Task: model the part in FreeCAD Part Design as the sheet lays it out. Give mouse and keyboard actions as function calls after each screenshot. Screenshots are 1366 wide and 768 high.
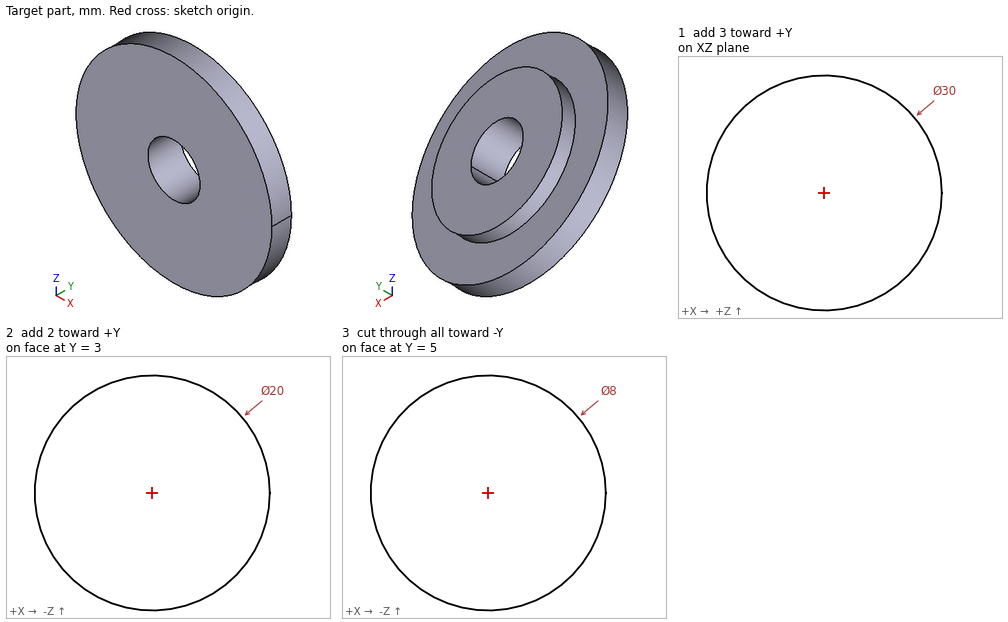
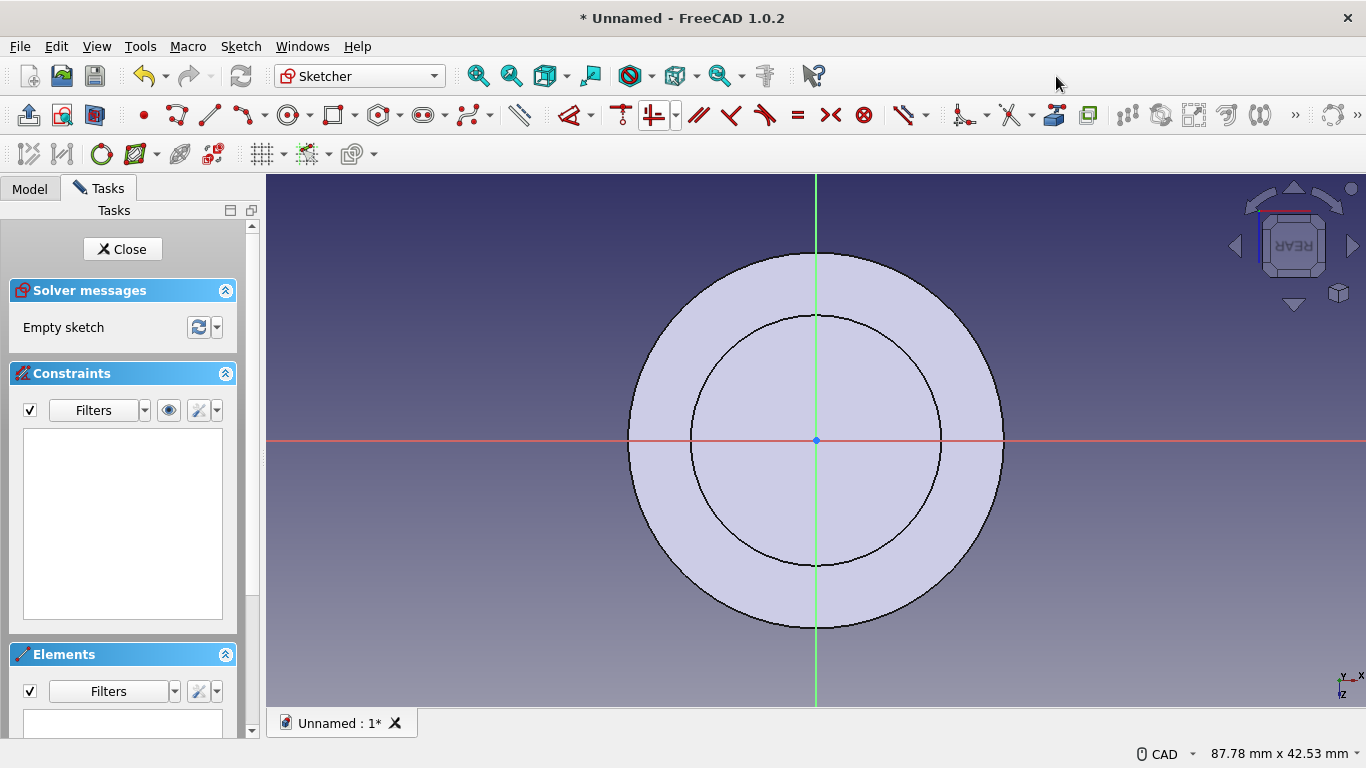
scroll(846, 440, up, 6)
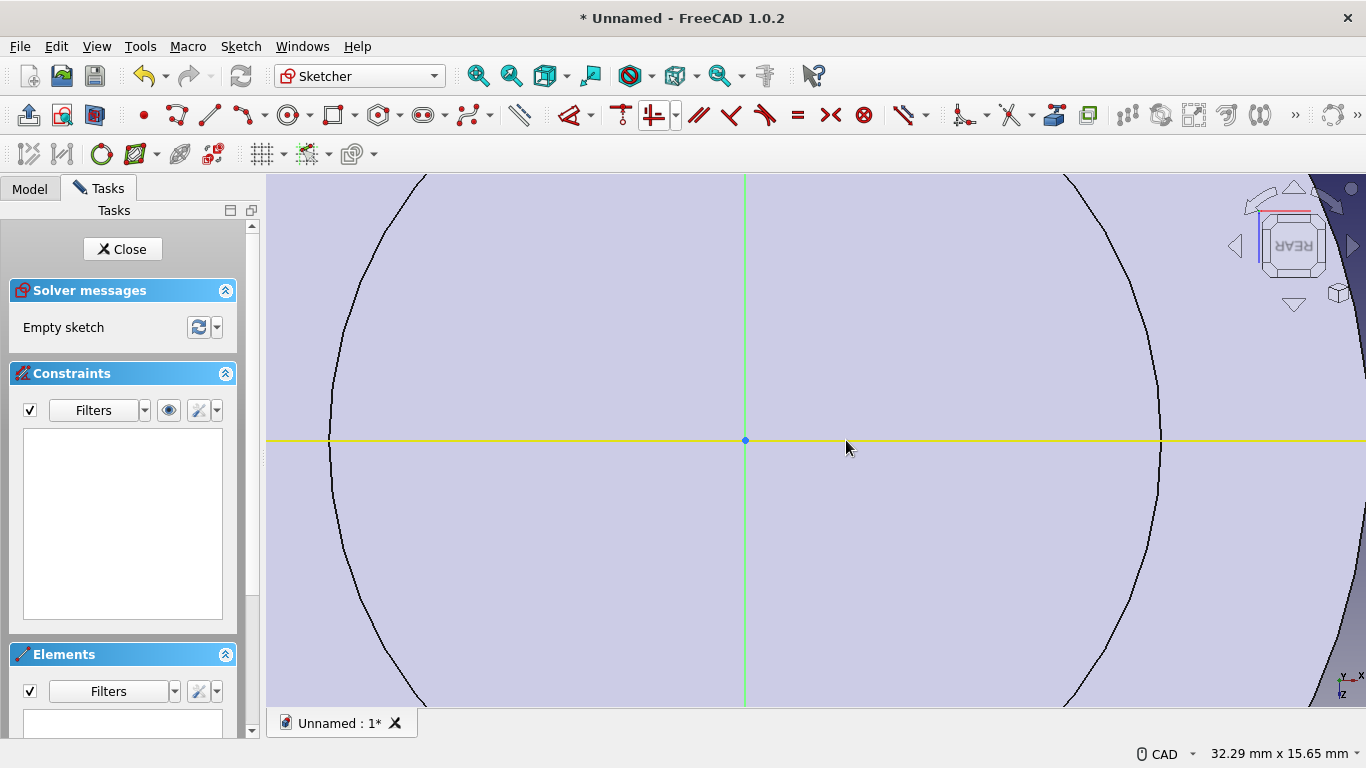
click(288, 116)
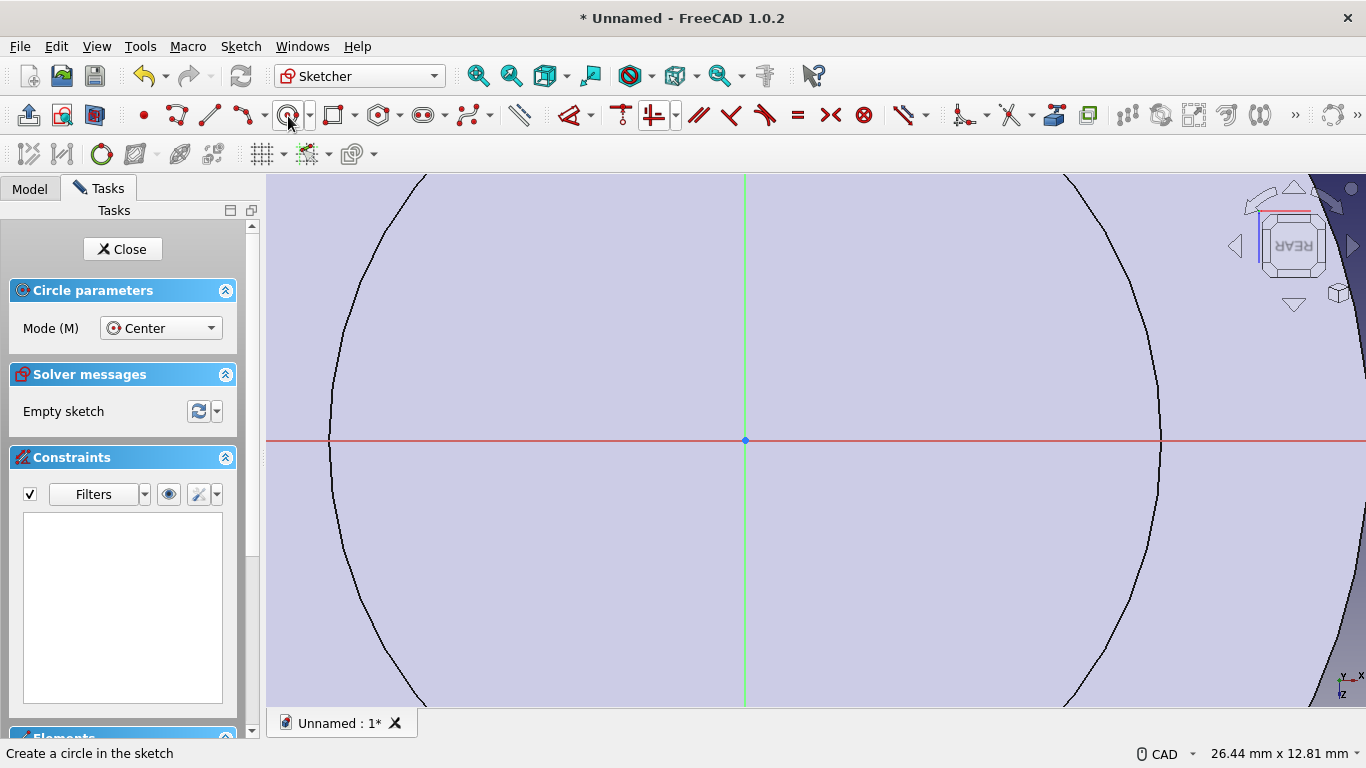
click(745, 440)
click(863, 323)
key(Escape)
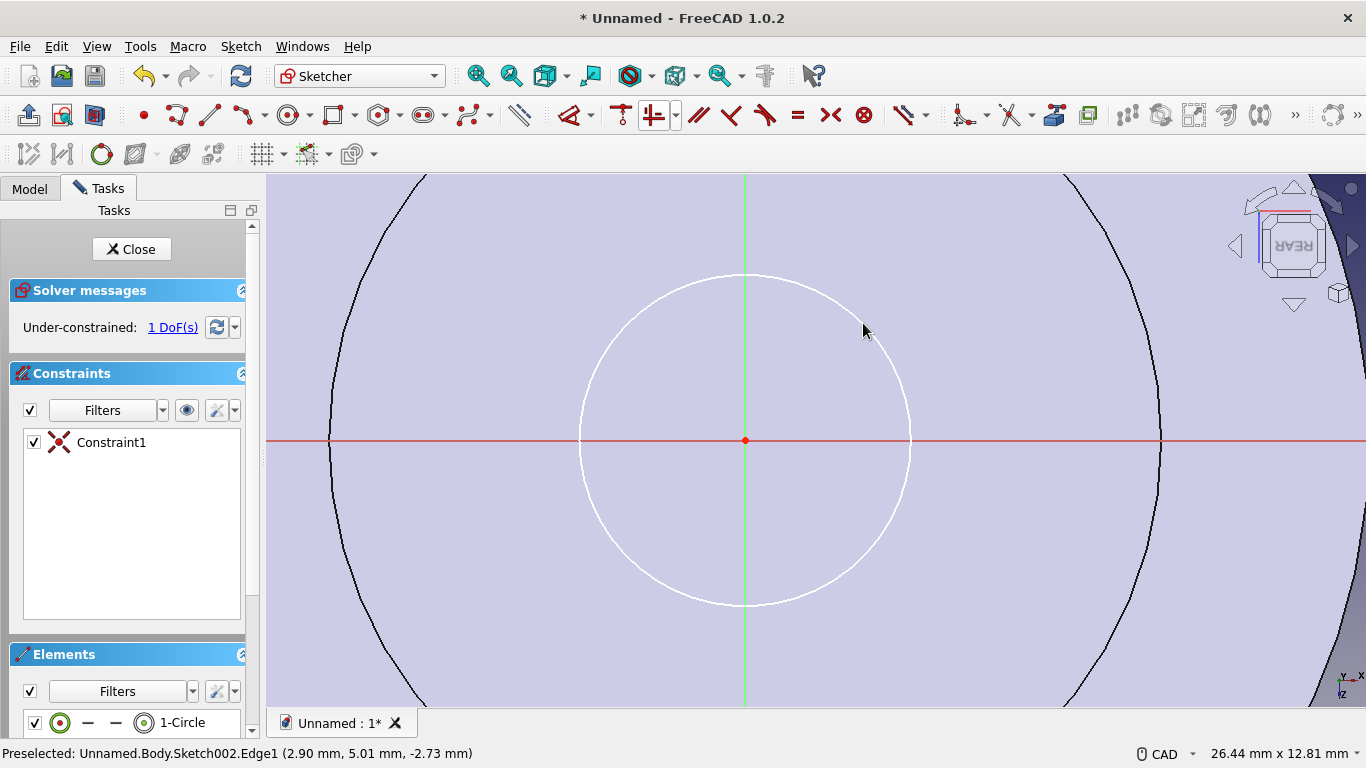
click(568, 116)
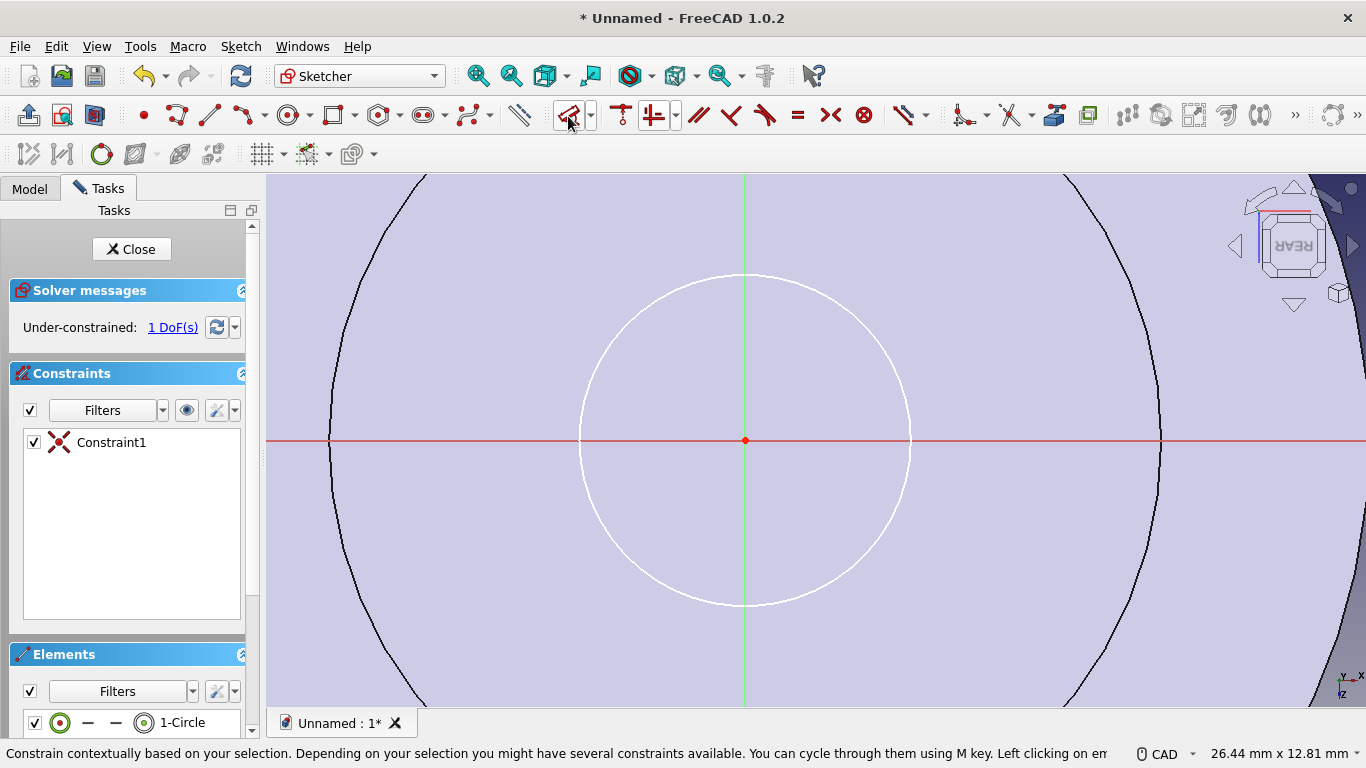
click(862, 323)
click(885, 300)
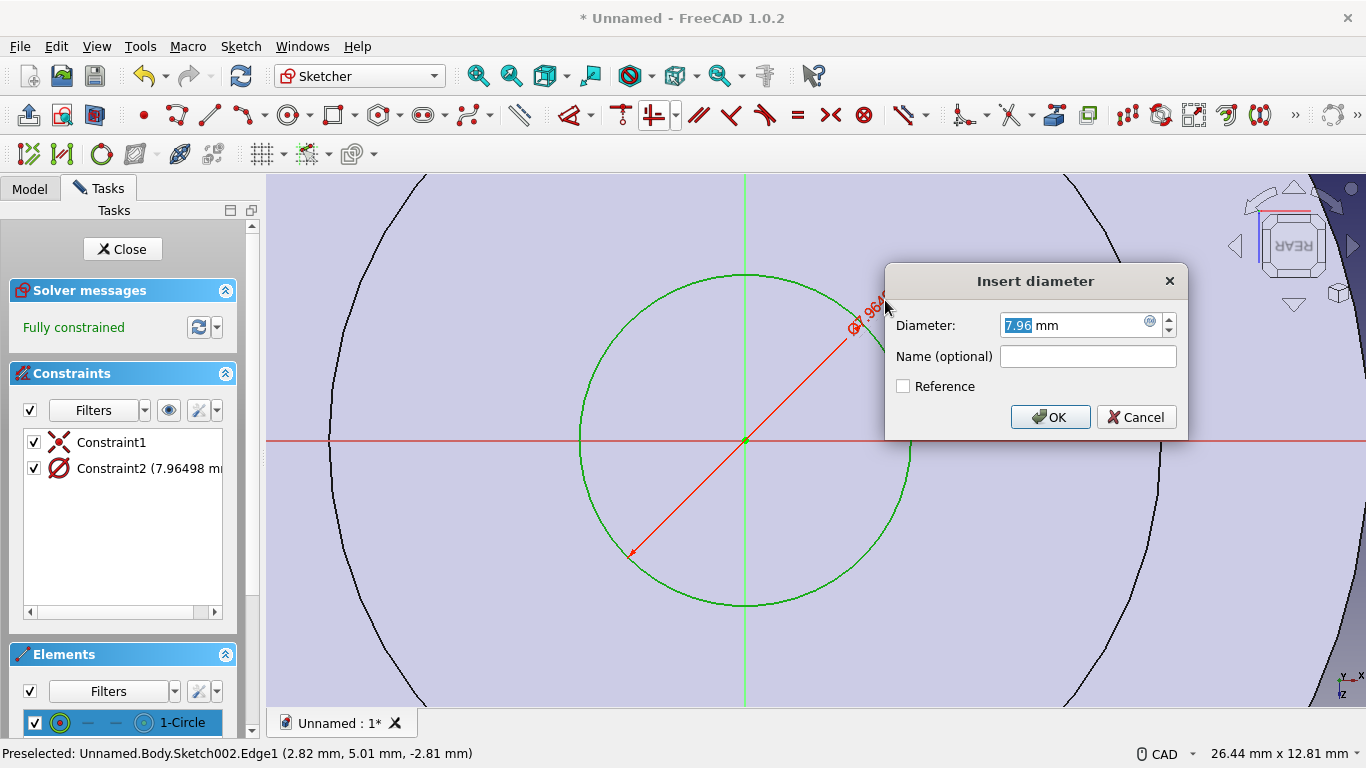
text(8)
key(Return)
key(Escape)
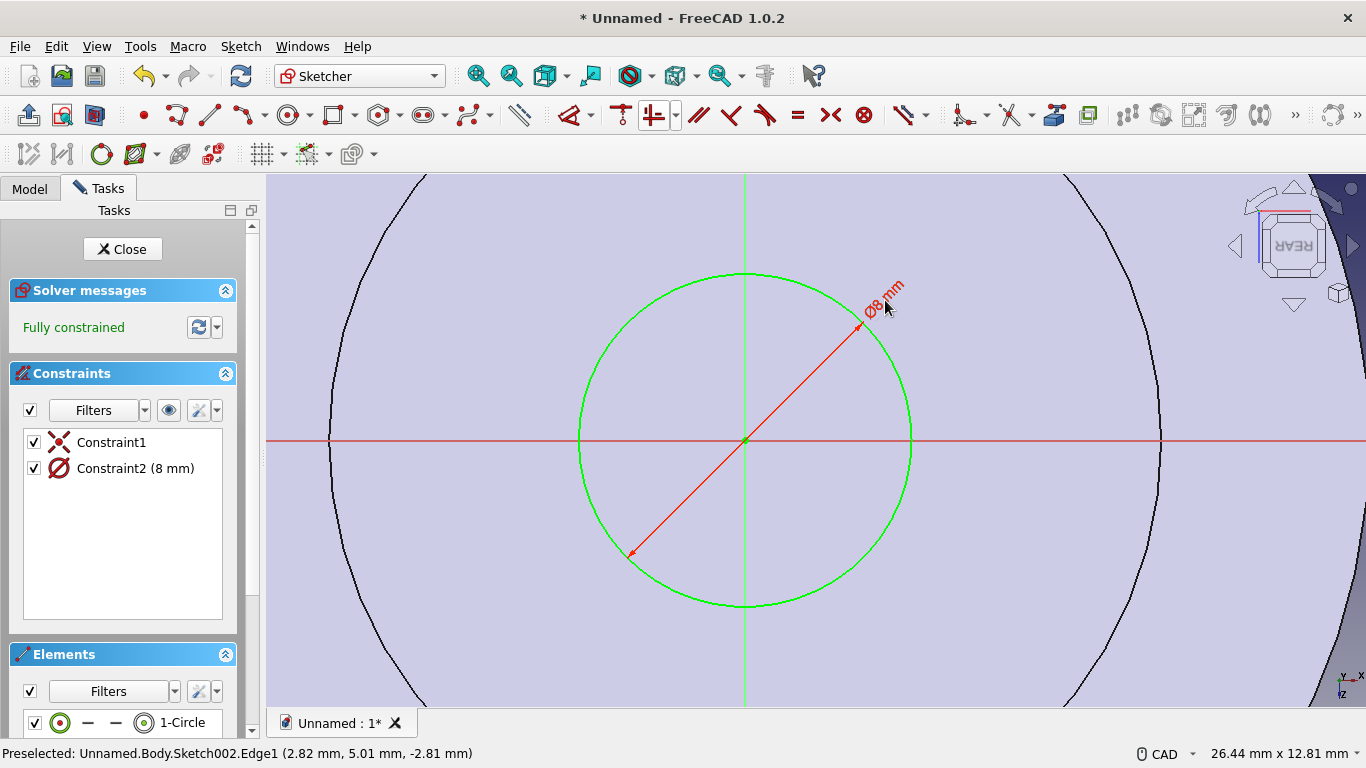
click(123, 249)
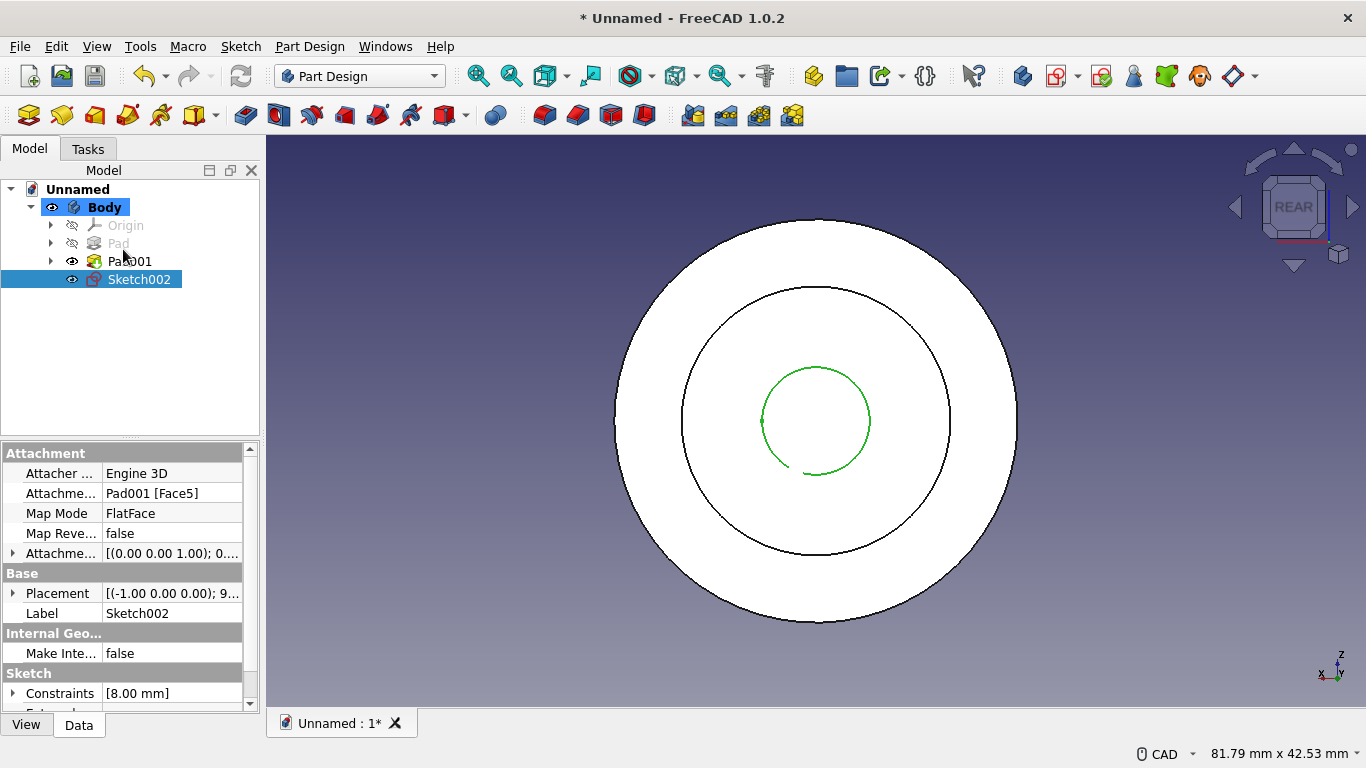
click(246, 116)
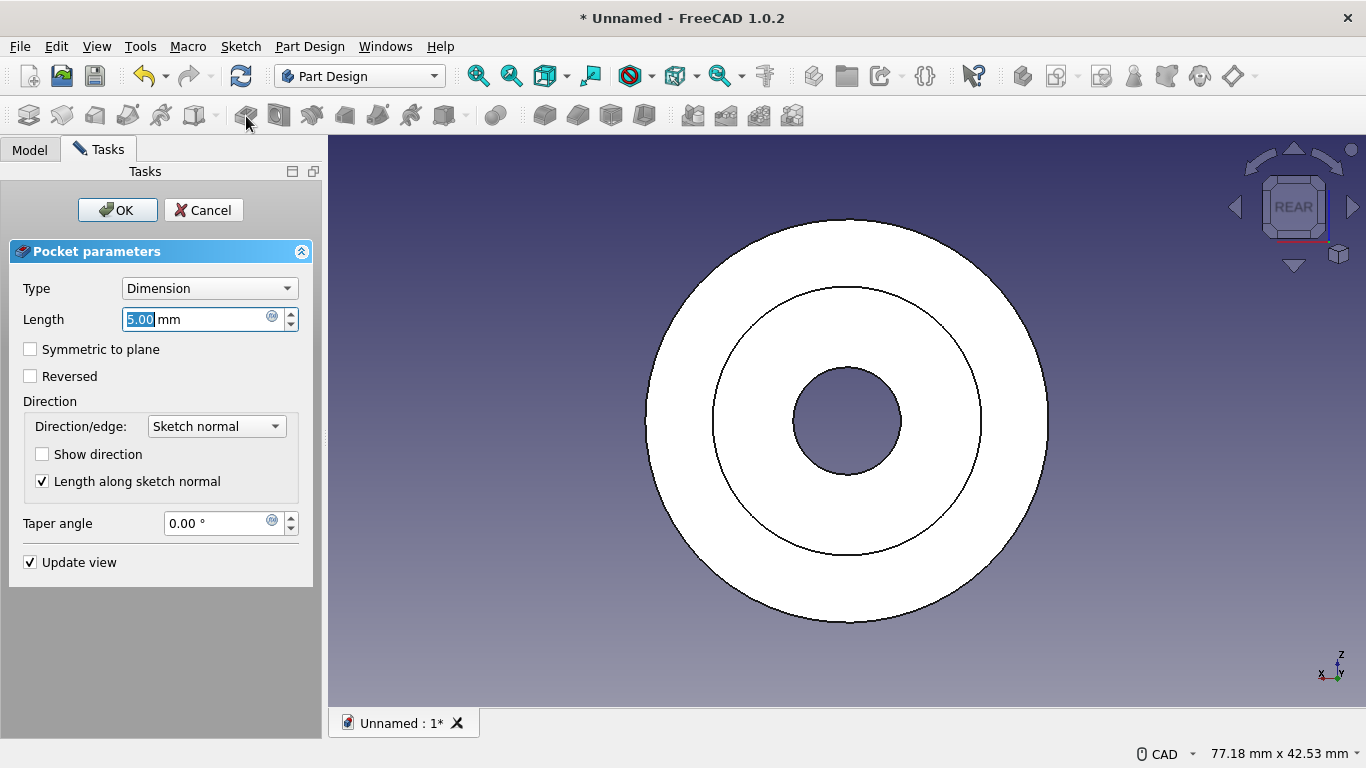
click(210, 288)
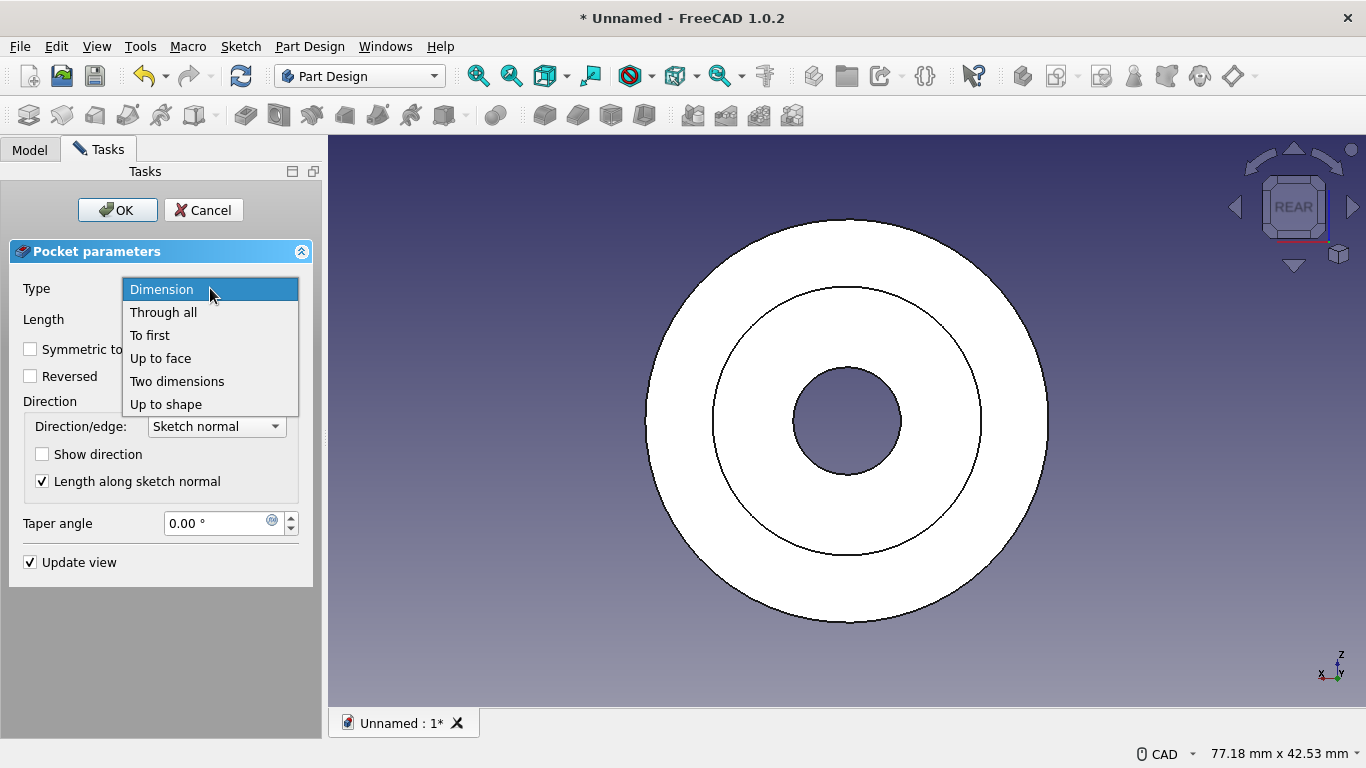
click(208, 312)